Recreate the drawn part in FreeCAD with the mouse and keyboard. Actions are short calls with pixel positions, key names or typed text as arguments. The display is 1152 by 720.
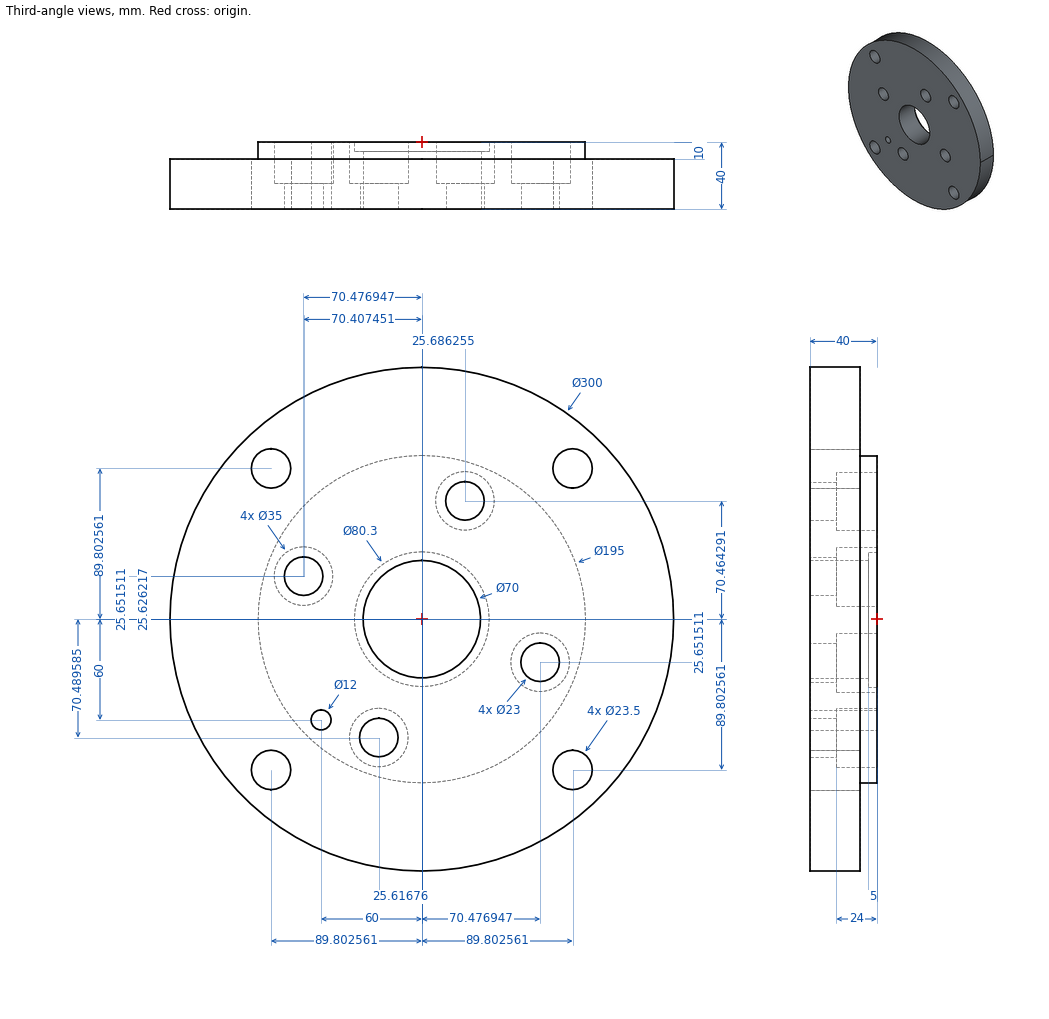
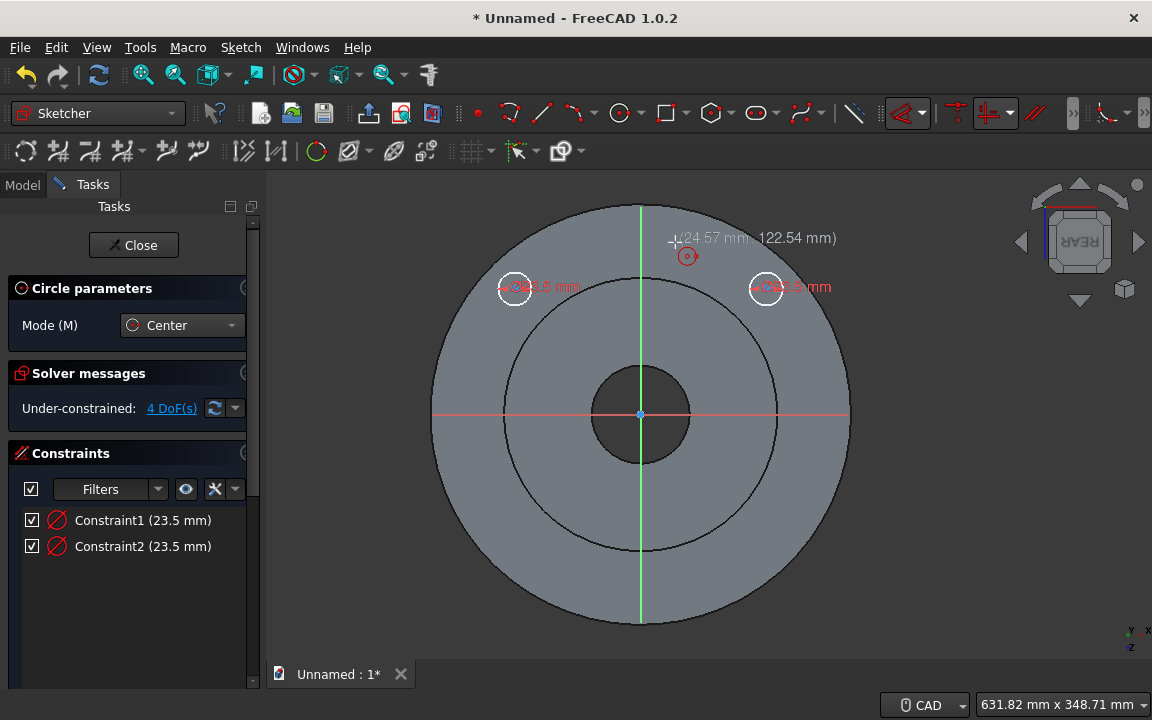
scroll(515, 540, up, 2)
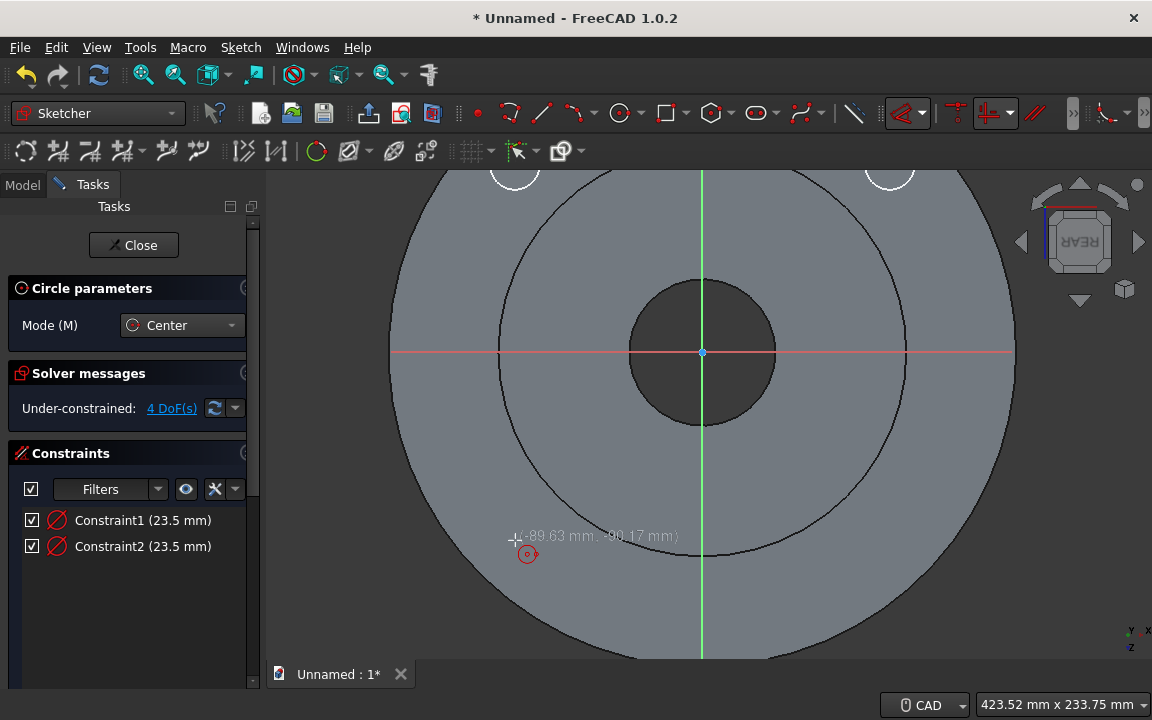
click(515, 540)
move(532, 523)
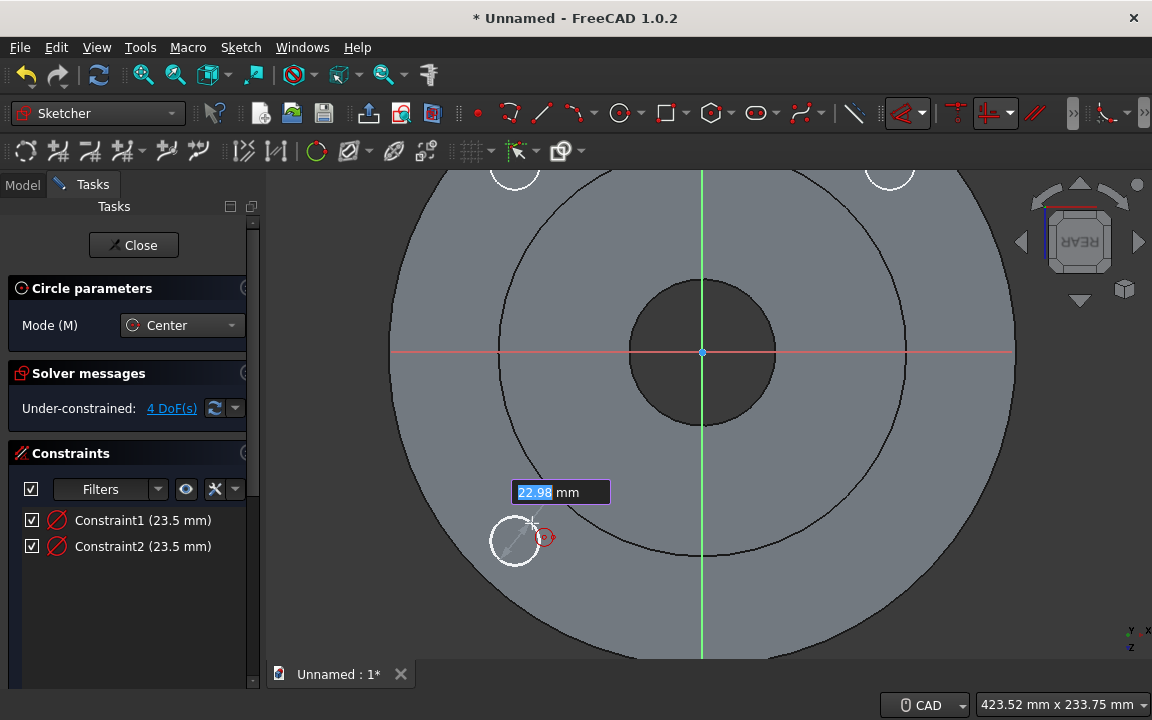
text(23.5)
key(Return)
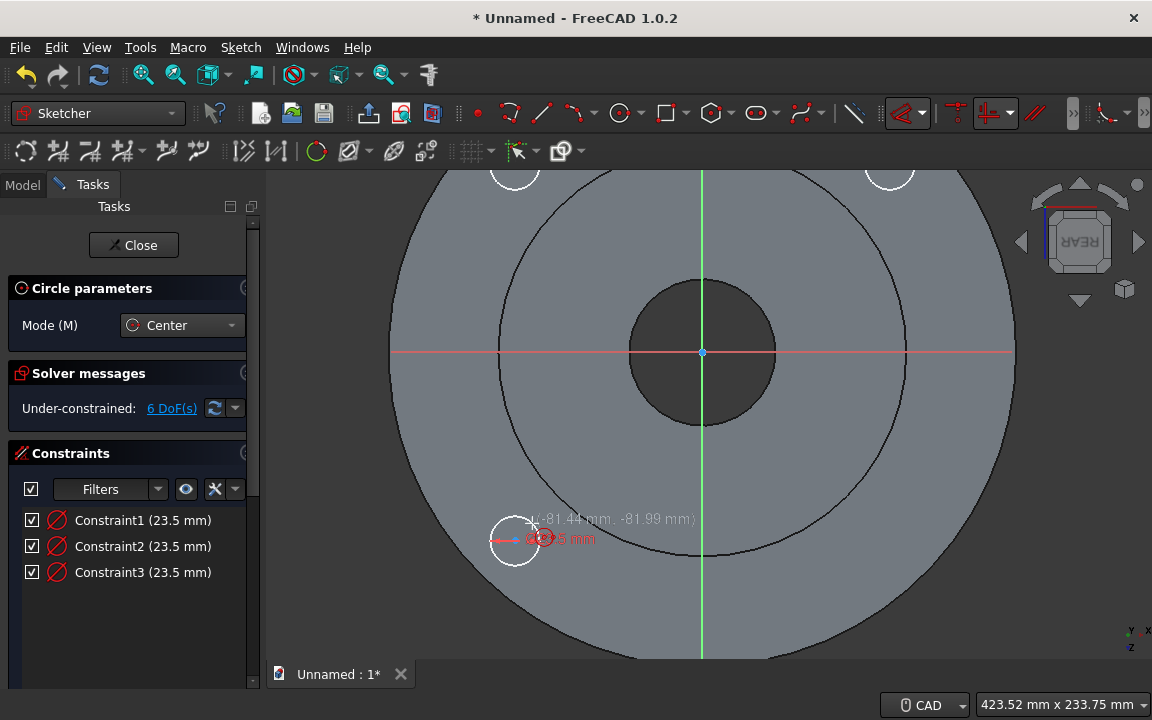
click(890, 540)
move(908, 523)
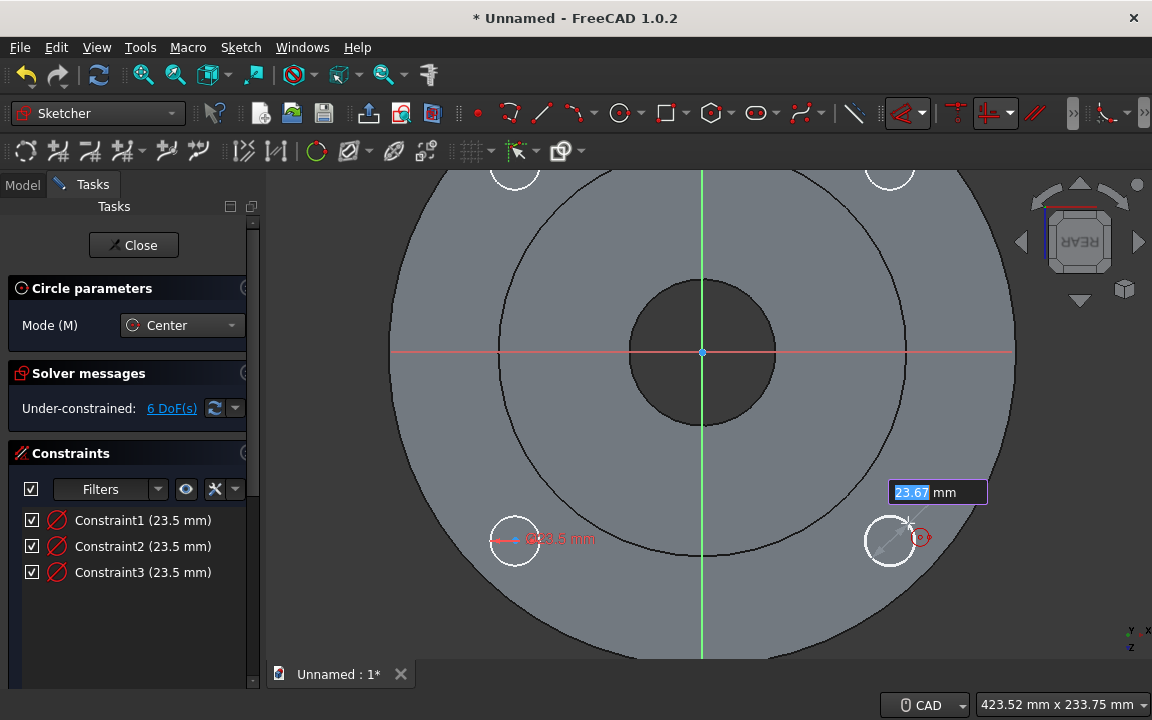
text(23.5)
key(Return)
key(Escape)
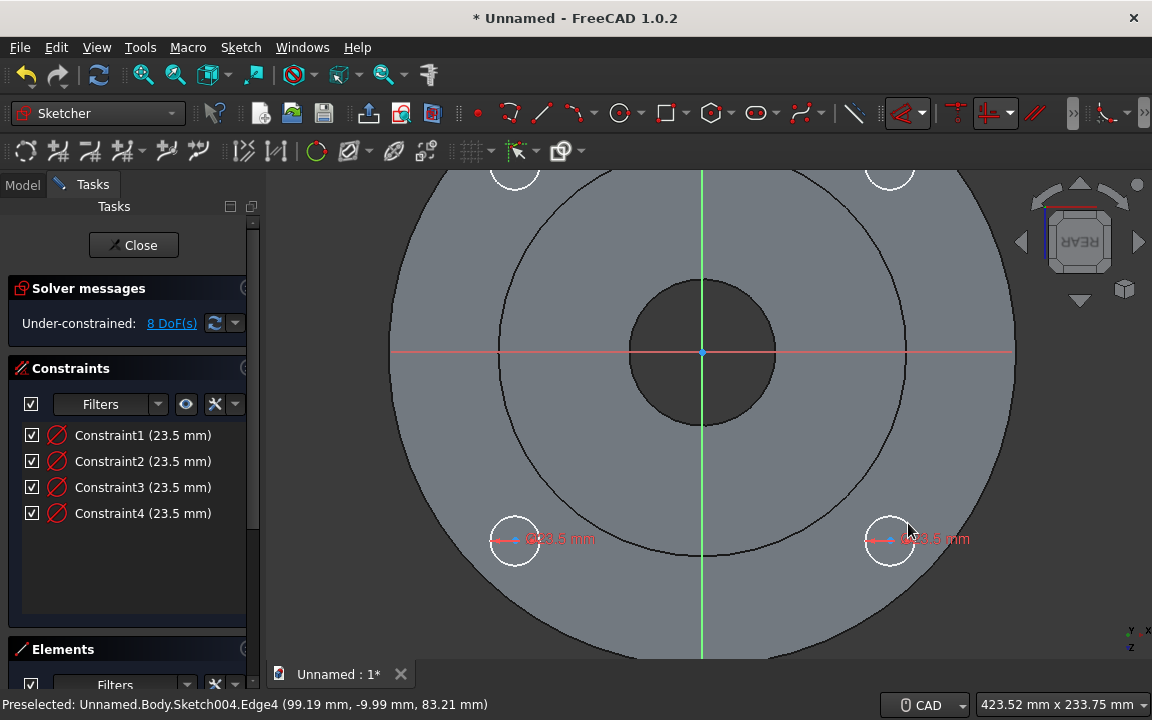
scroll(515, 541, down, 2)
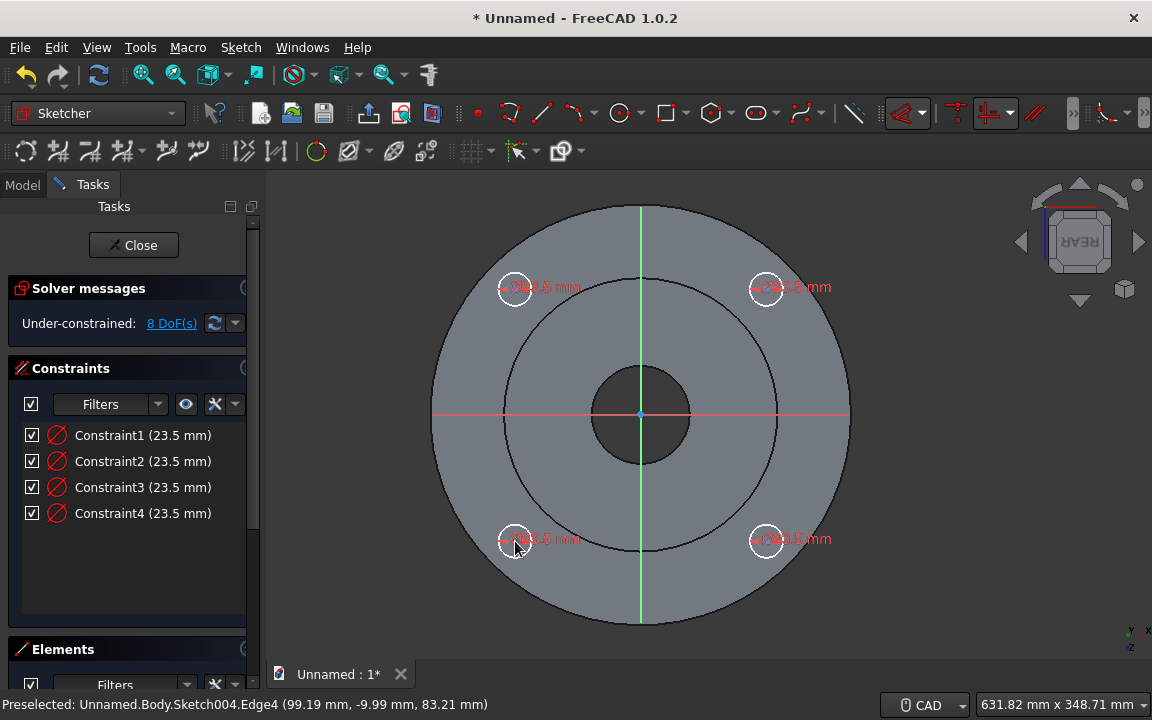
click(766, 289)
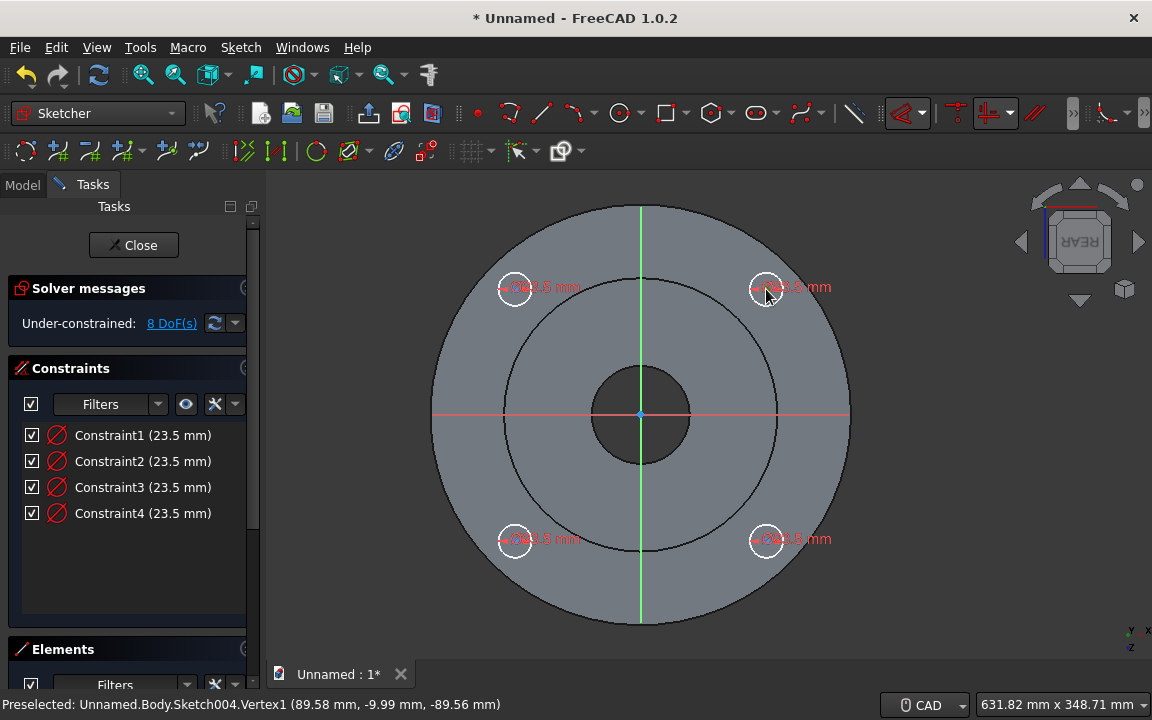
click(515, 289)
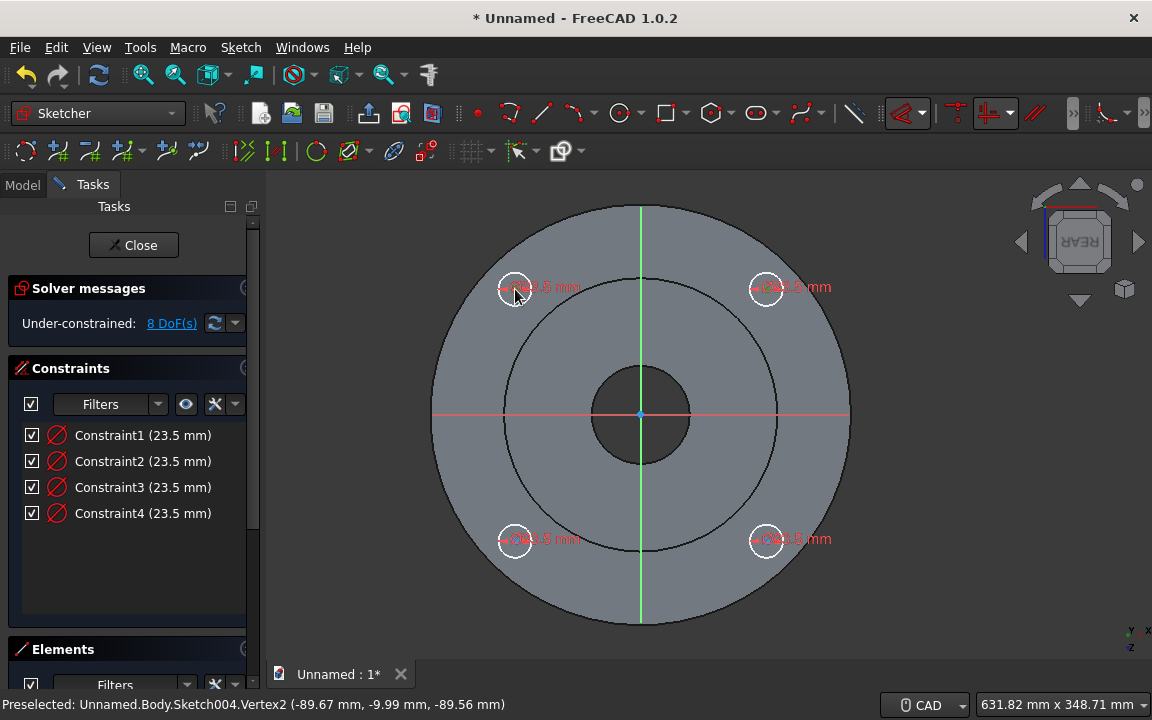
click(1012, 114)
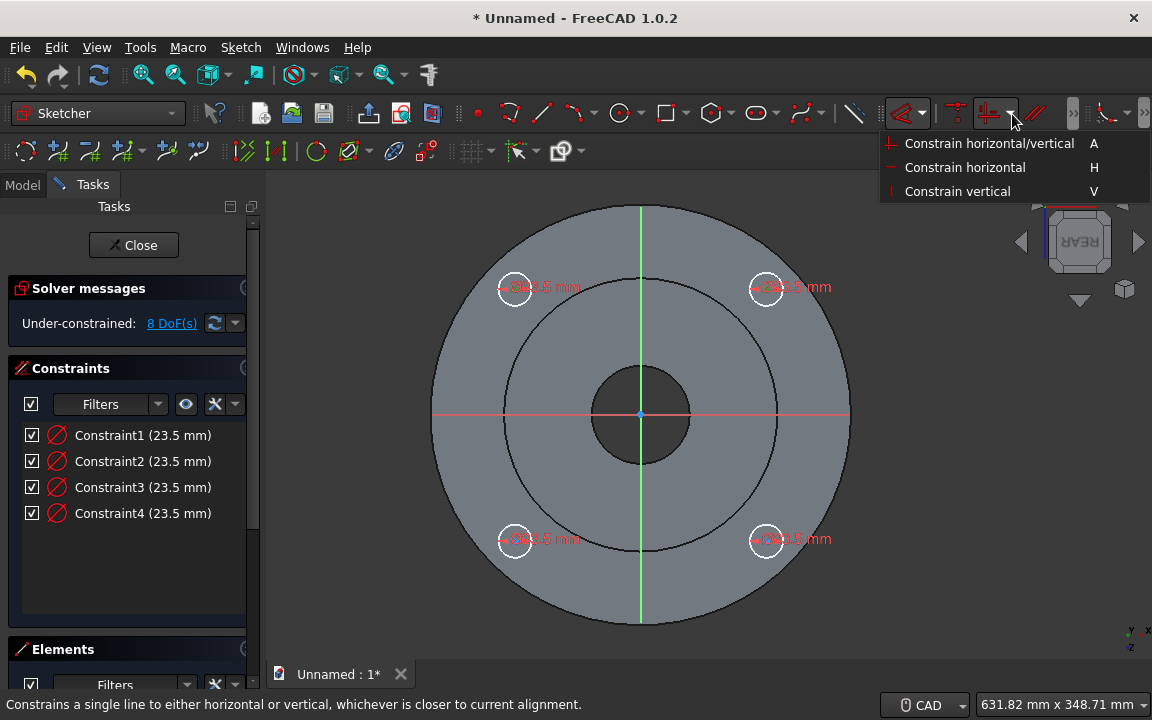
click(1015, 167)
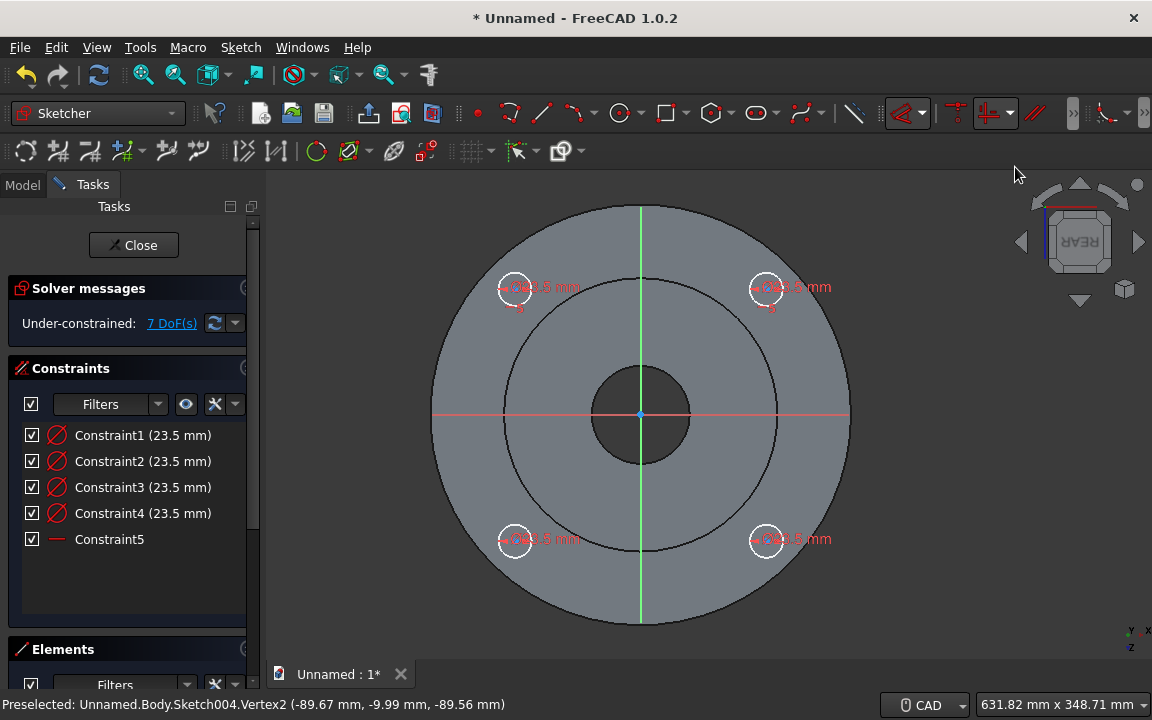
click(515, 289)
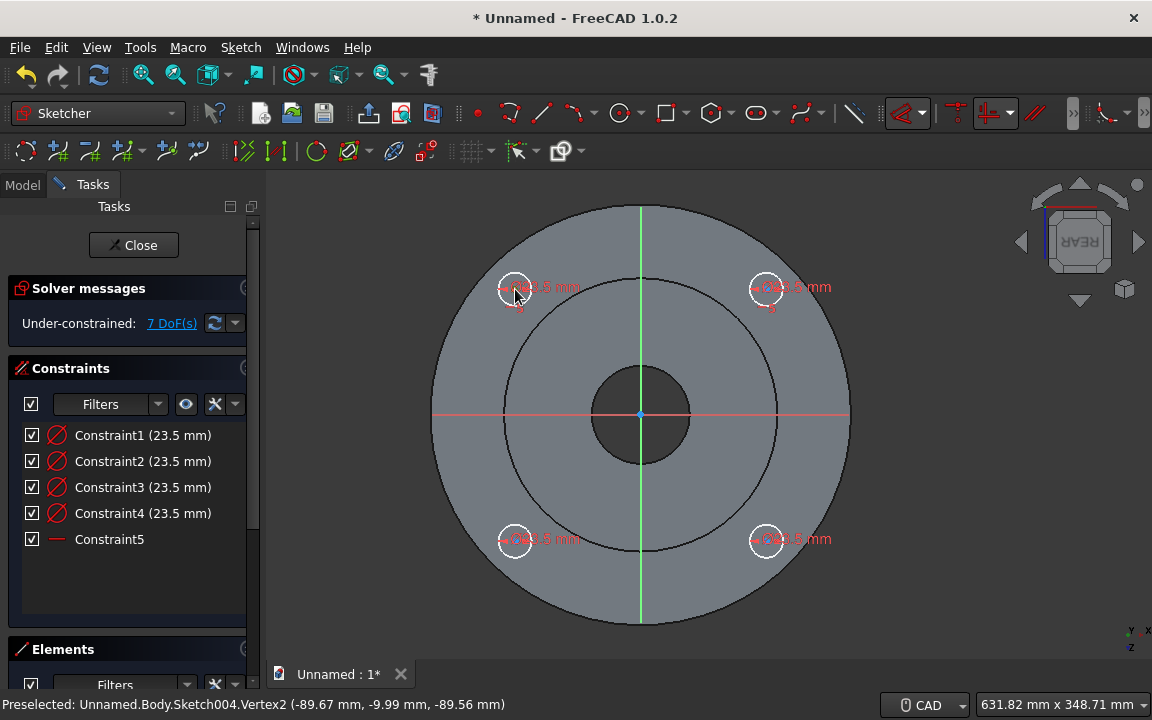
click(515, 541)